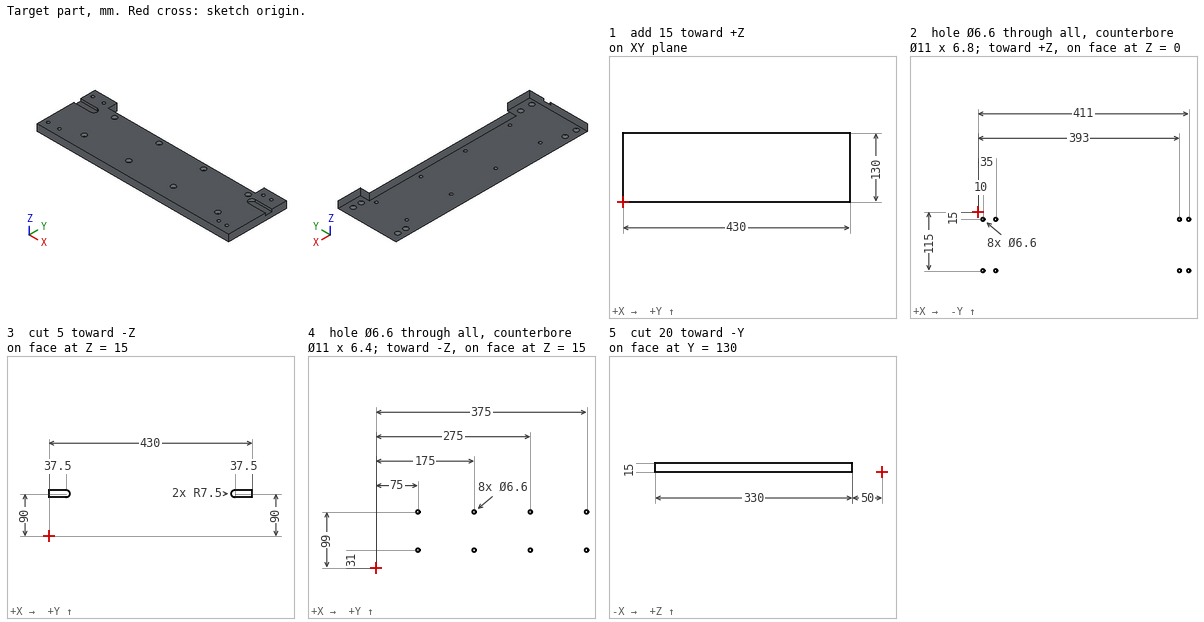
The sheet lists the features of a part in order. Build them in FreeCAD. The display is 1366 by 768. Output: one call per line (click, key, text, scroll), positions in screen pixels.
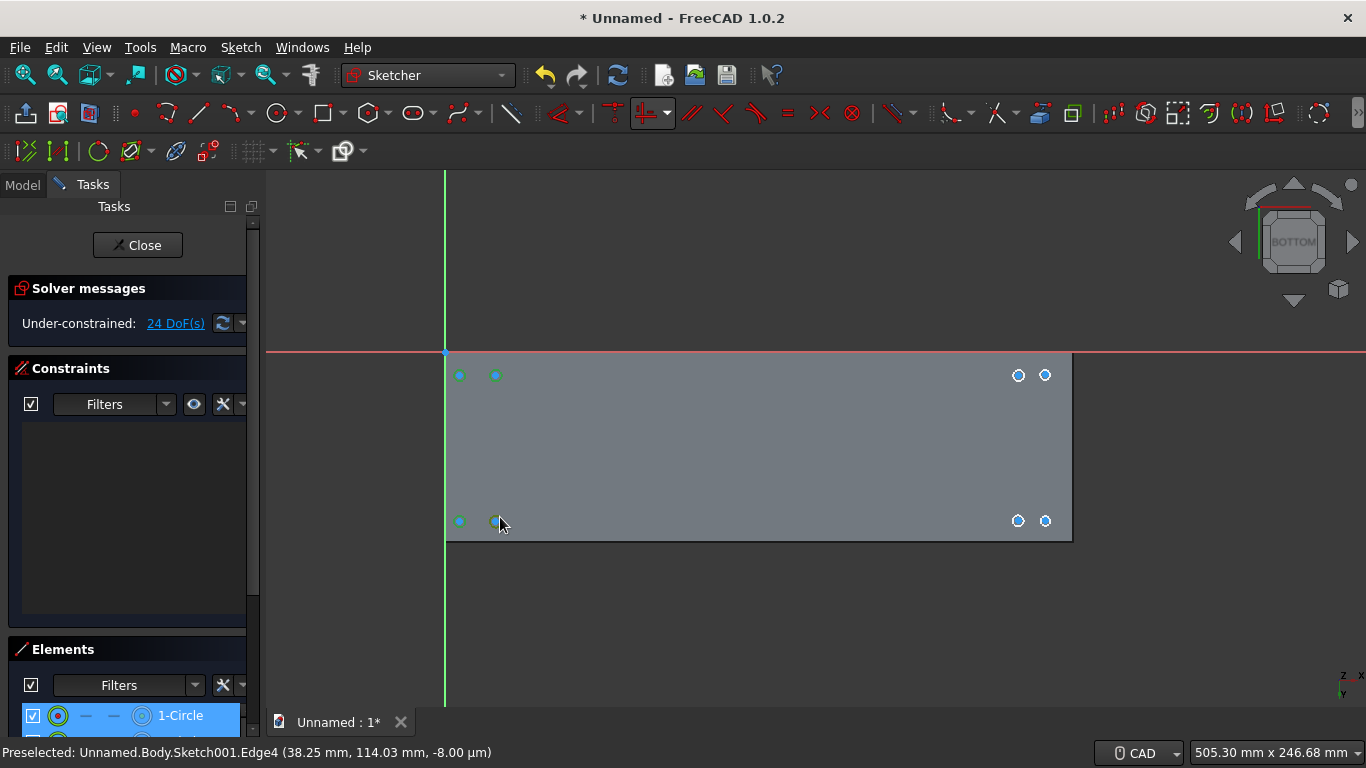
scroll(1023, 372, up, 5)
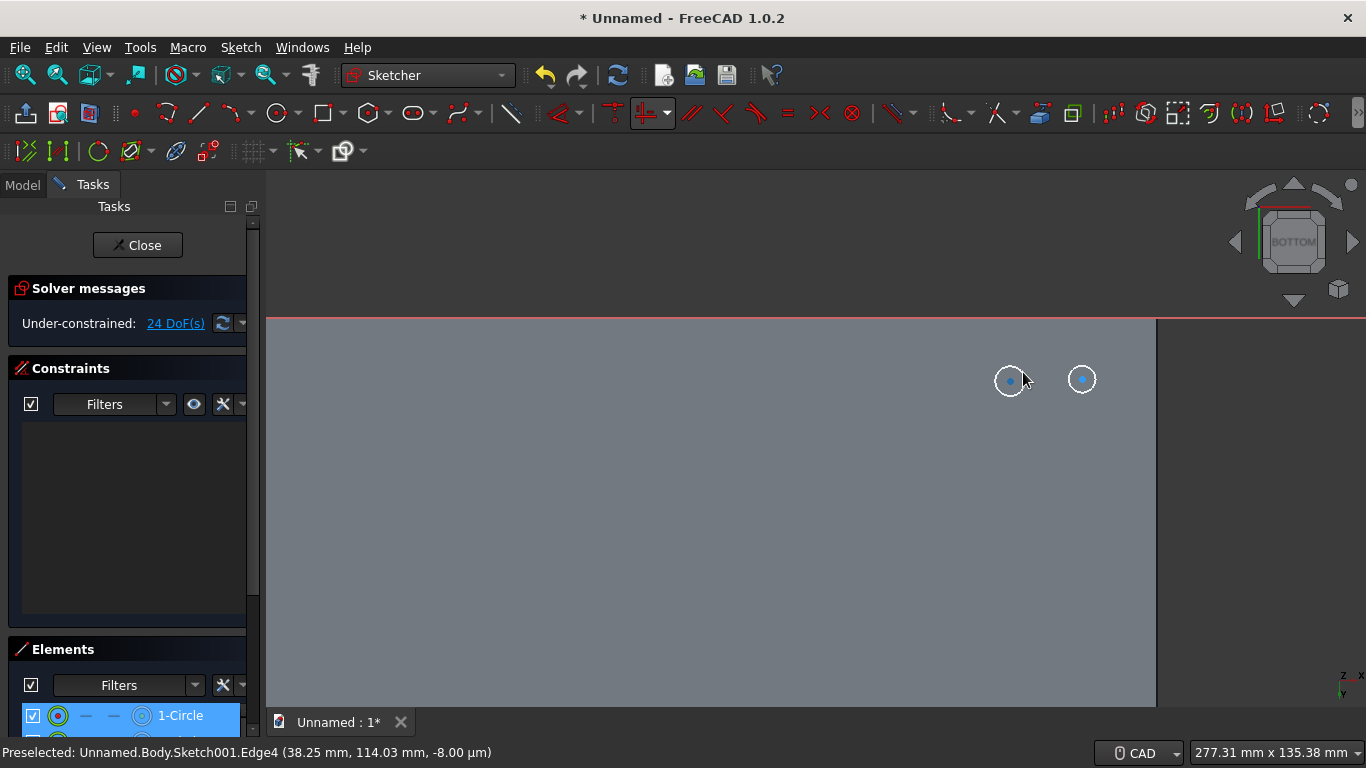
click(1021, 371)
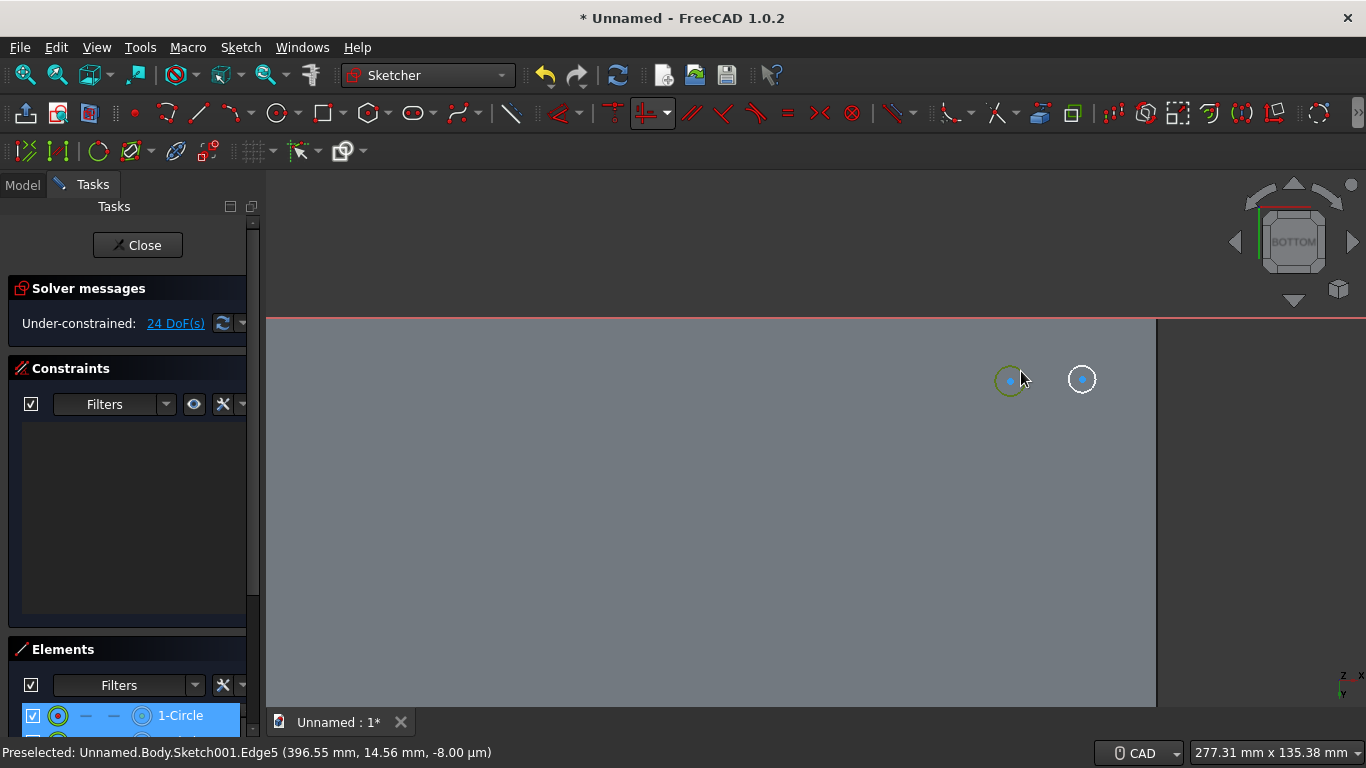
click(1092, 370)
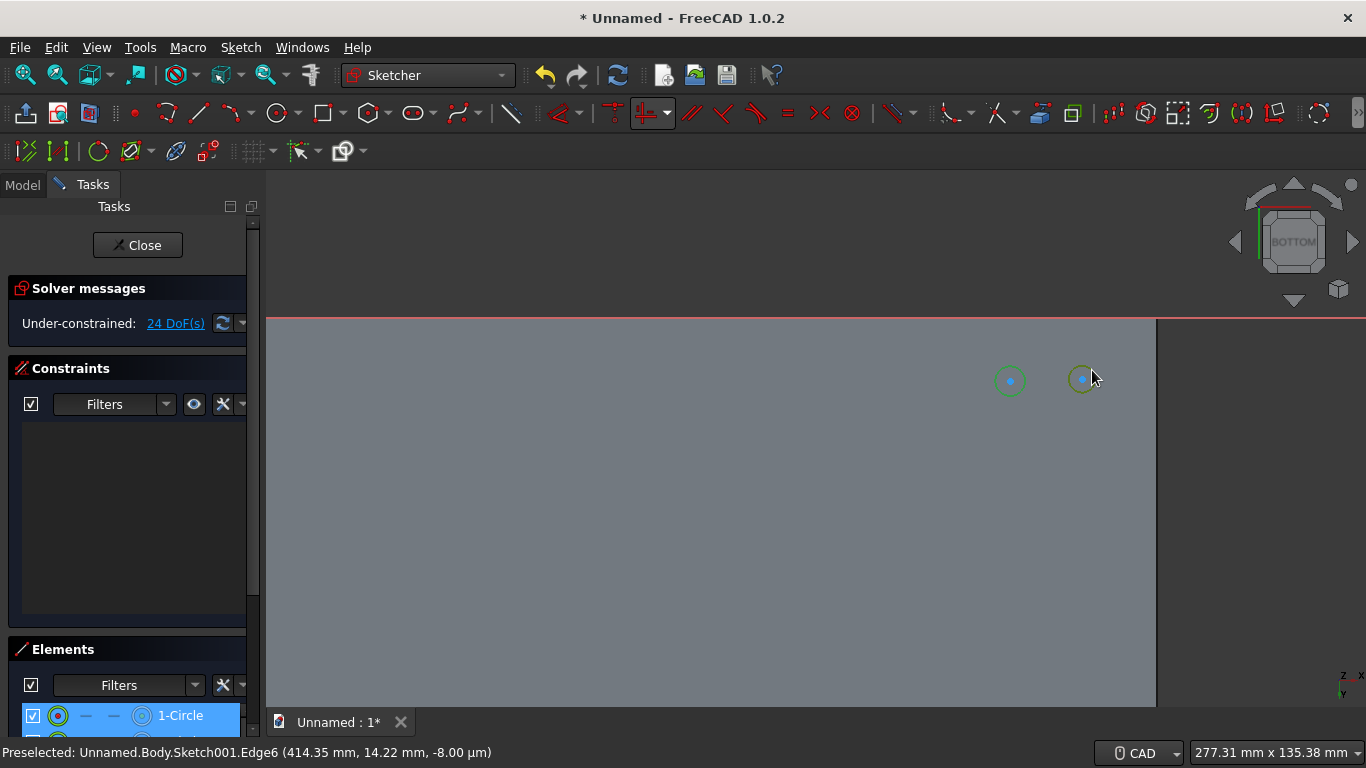
scroll(1024, 372, down, 5)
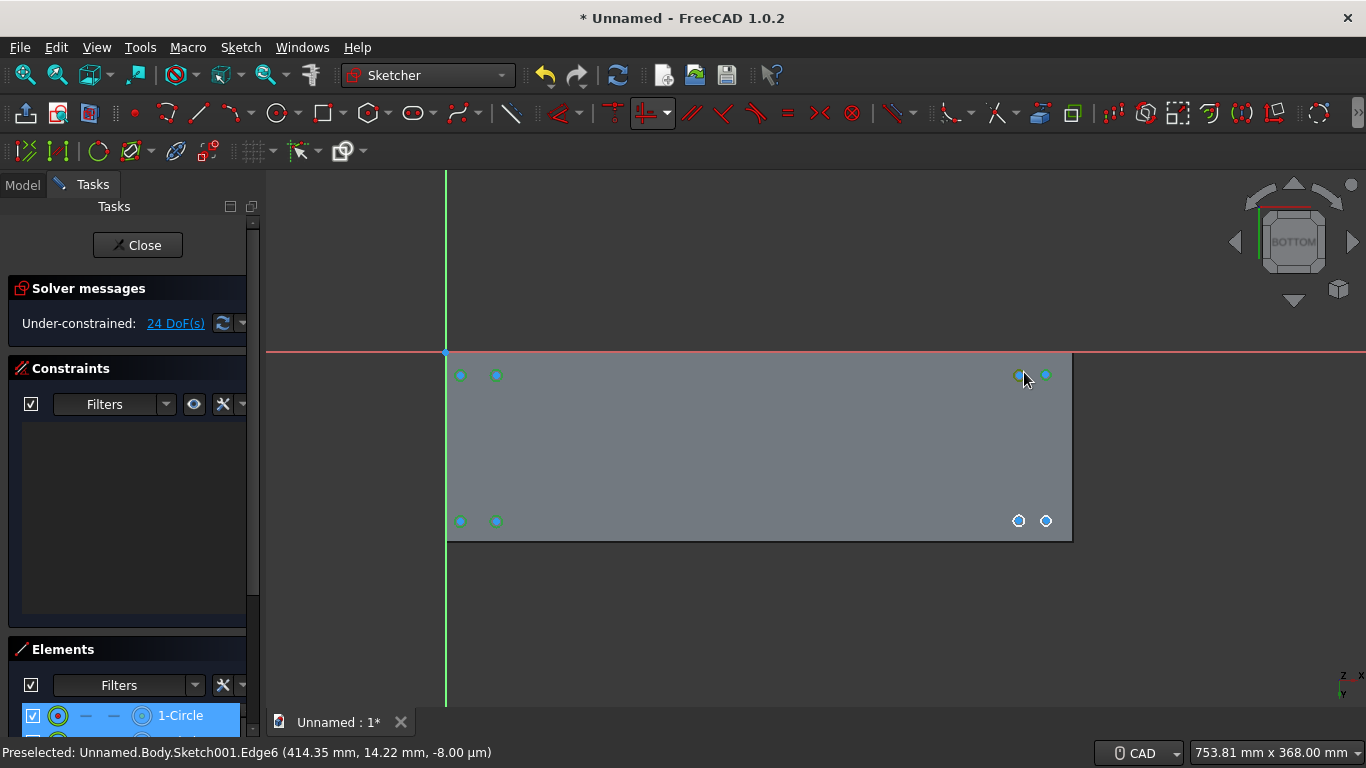
scroll(1023, 517, up, 5)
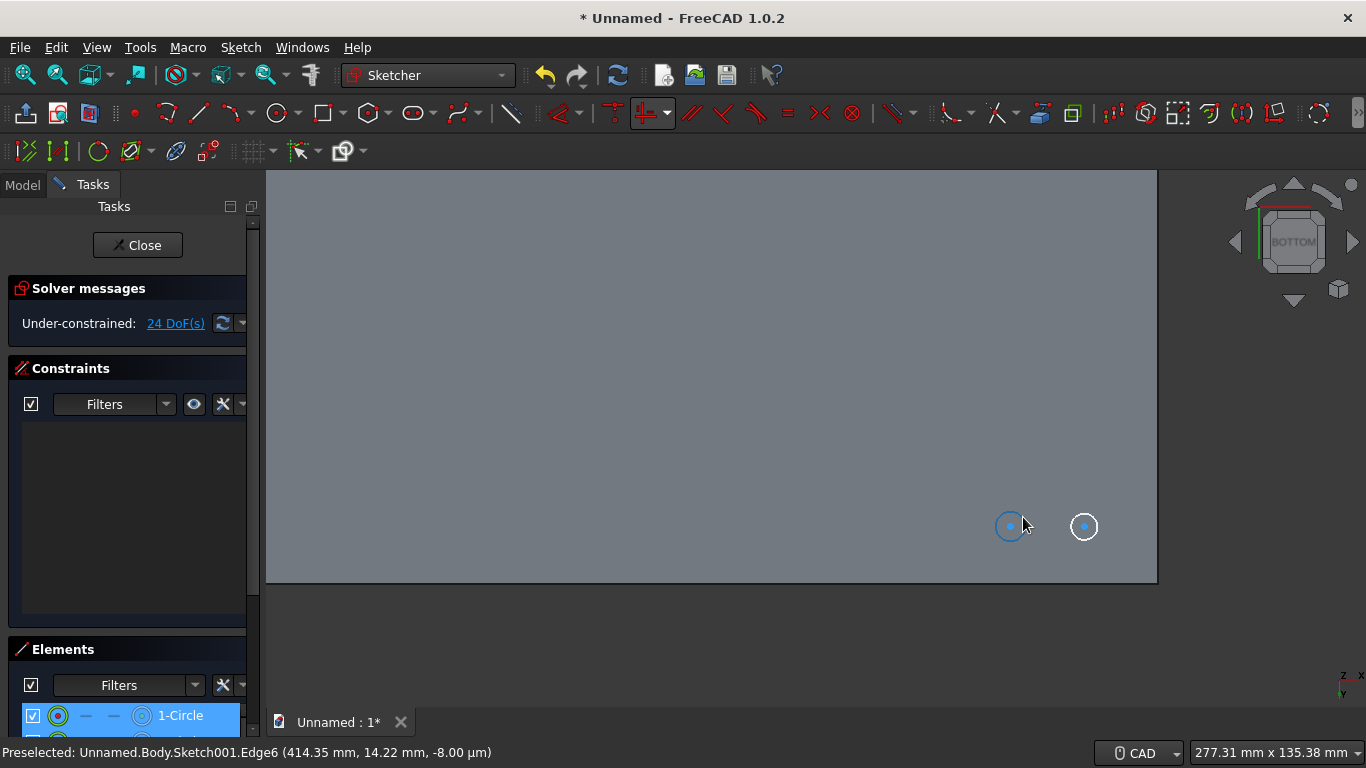
click(1021, 516)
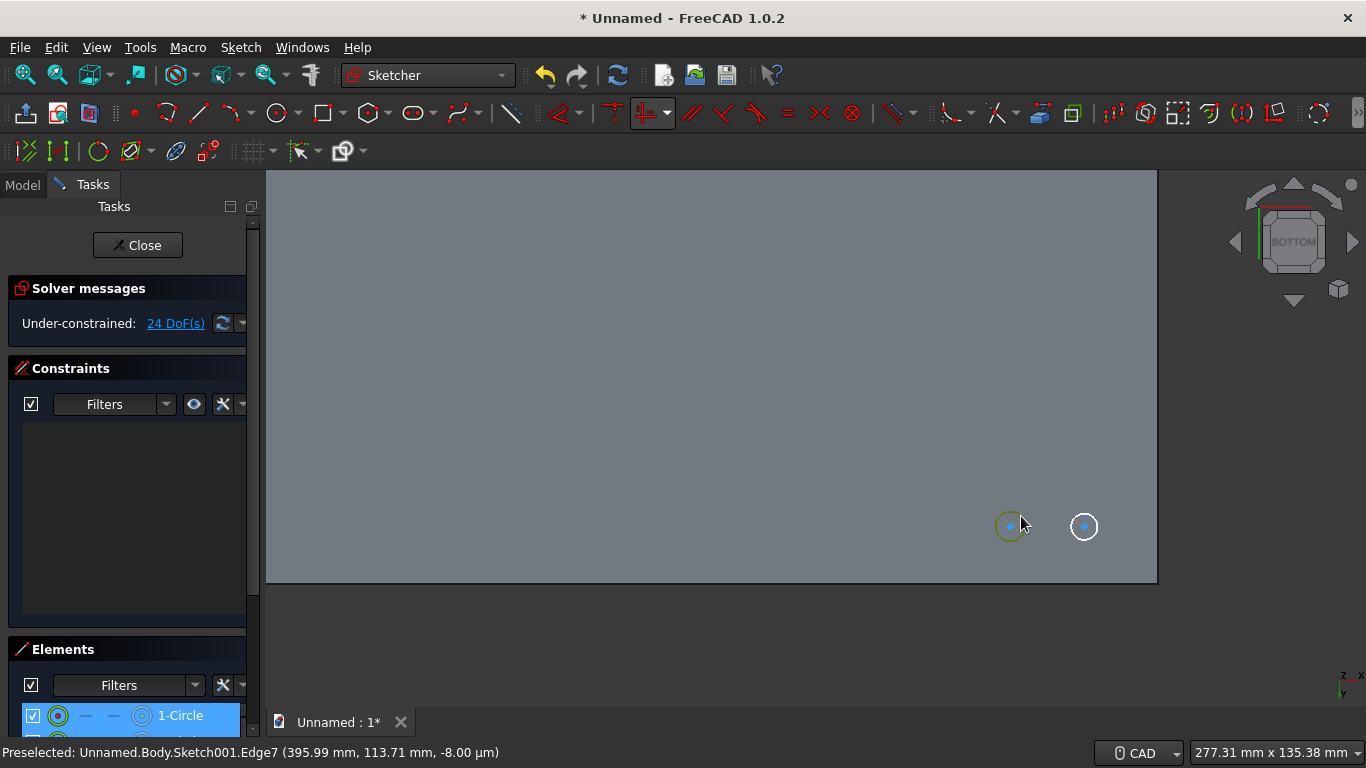
click(1094, 517)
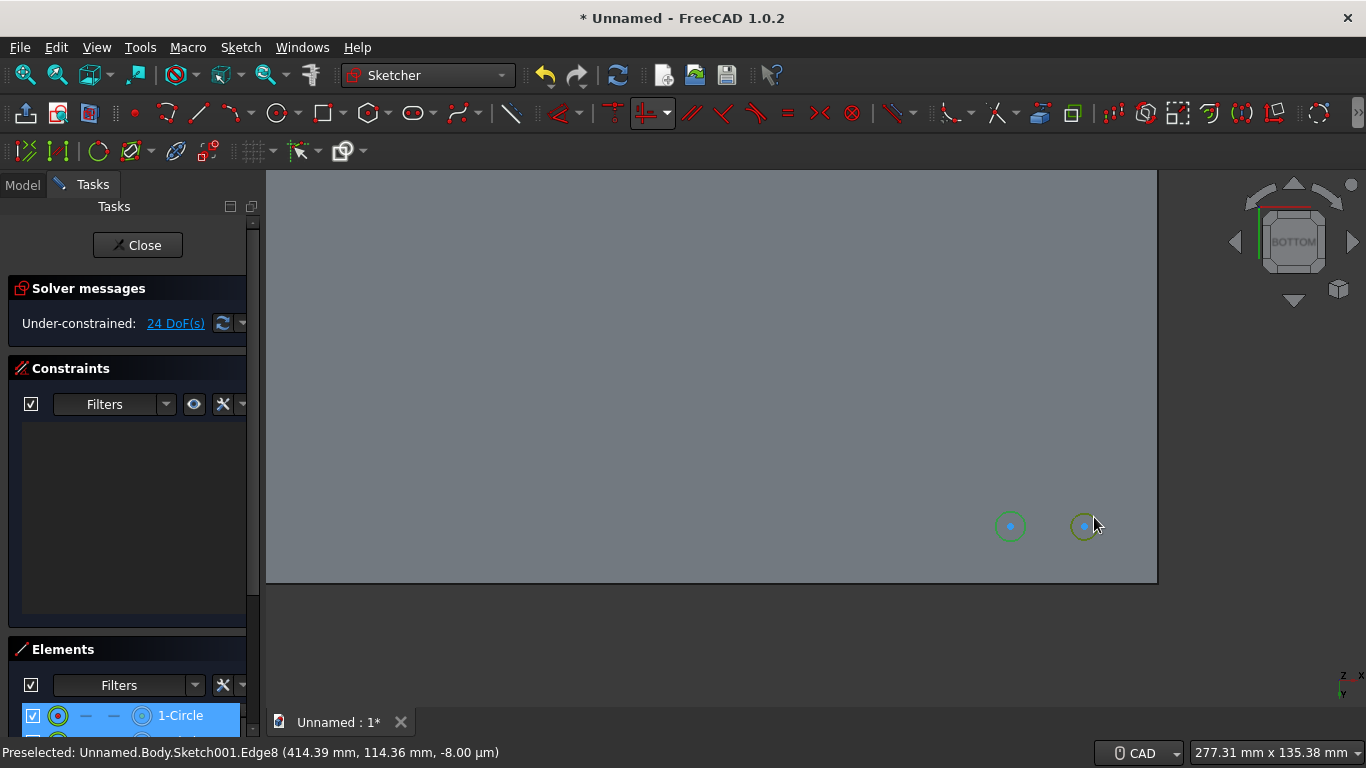
key(e)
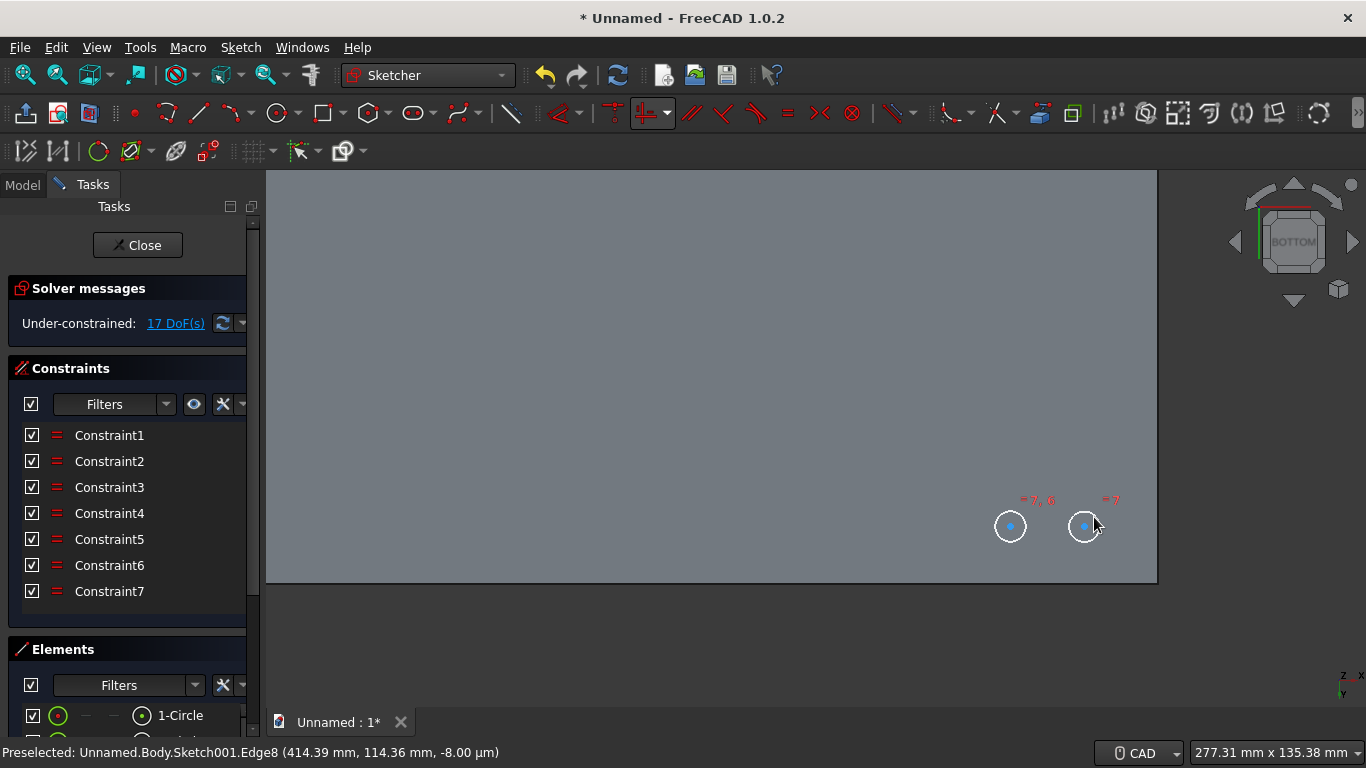
scroll(1023, 517, down, 5)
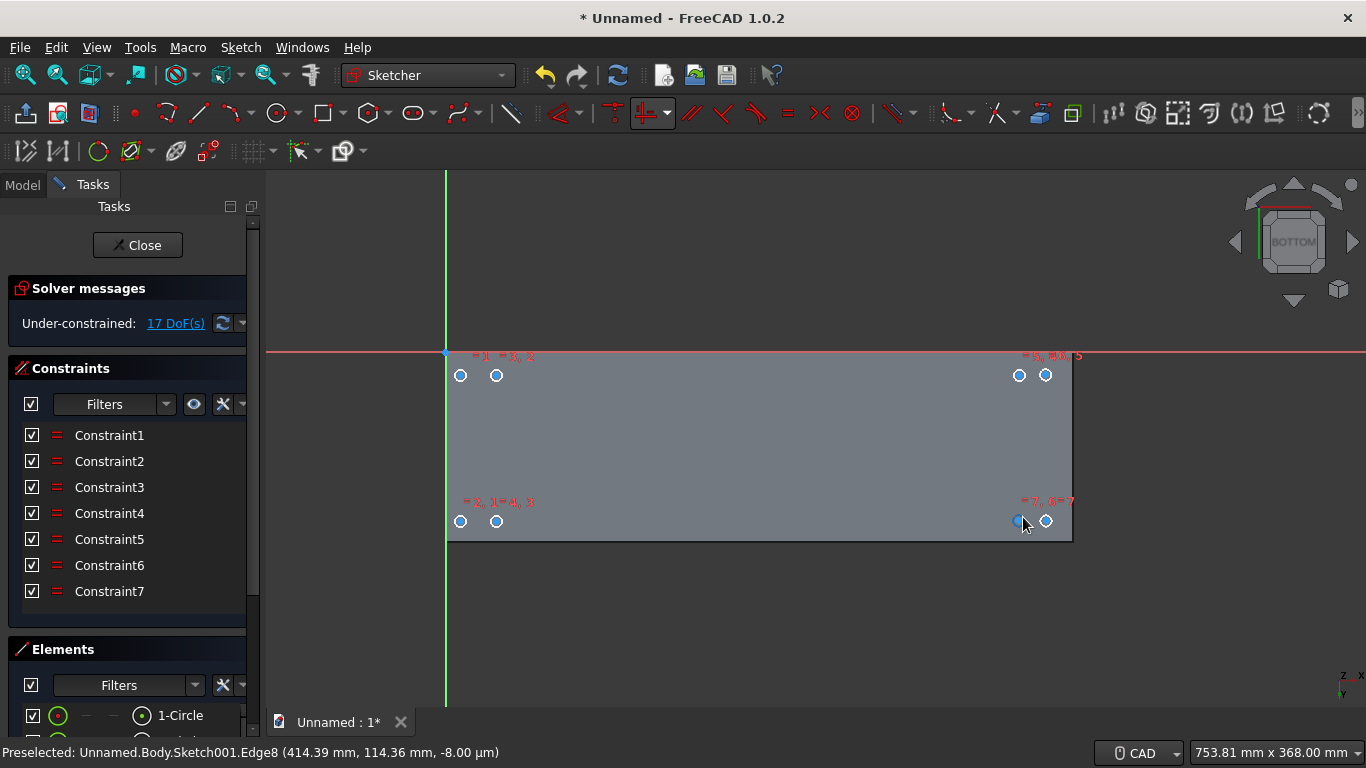
click(460, 376)